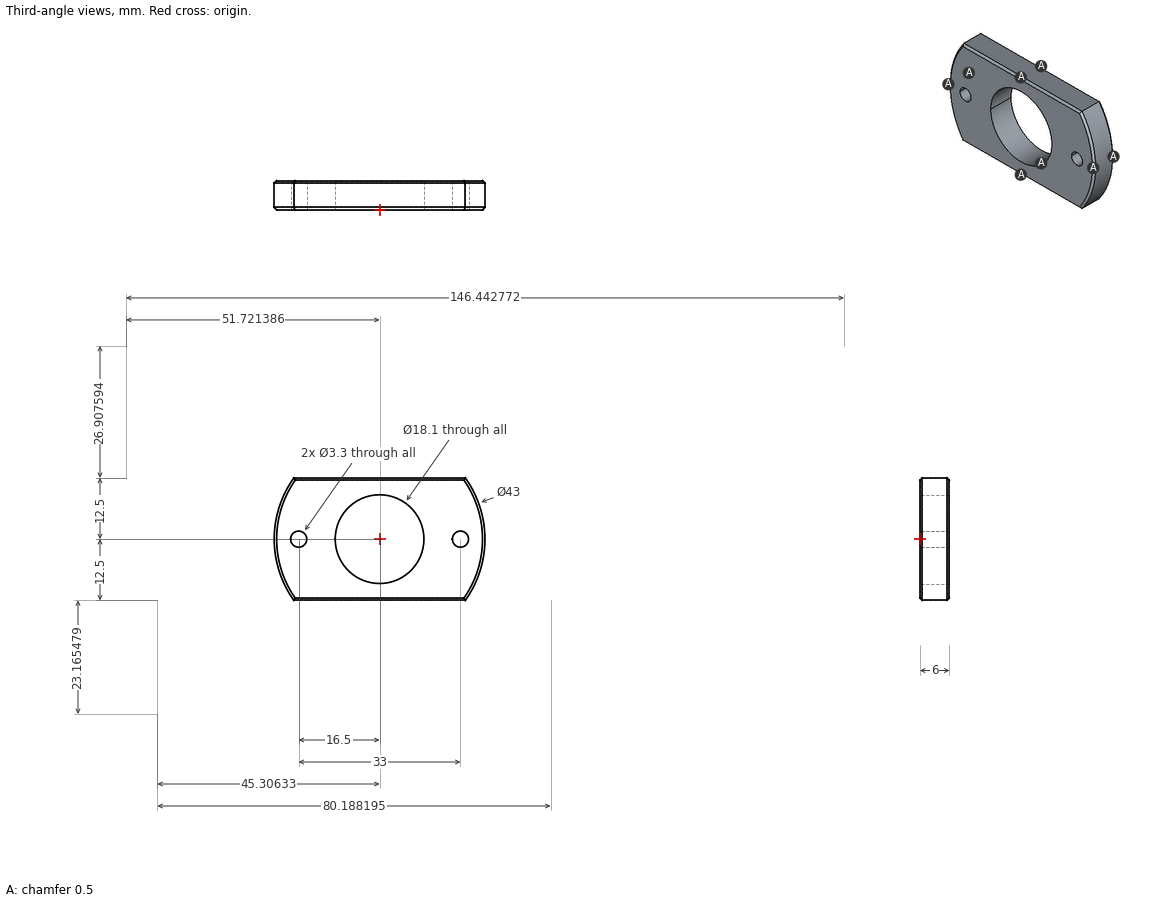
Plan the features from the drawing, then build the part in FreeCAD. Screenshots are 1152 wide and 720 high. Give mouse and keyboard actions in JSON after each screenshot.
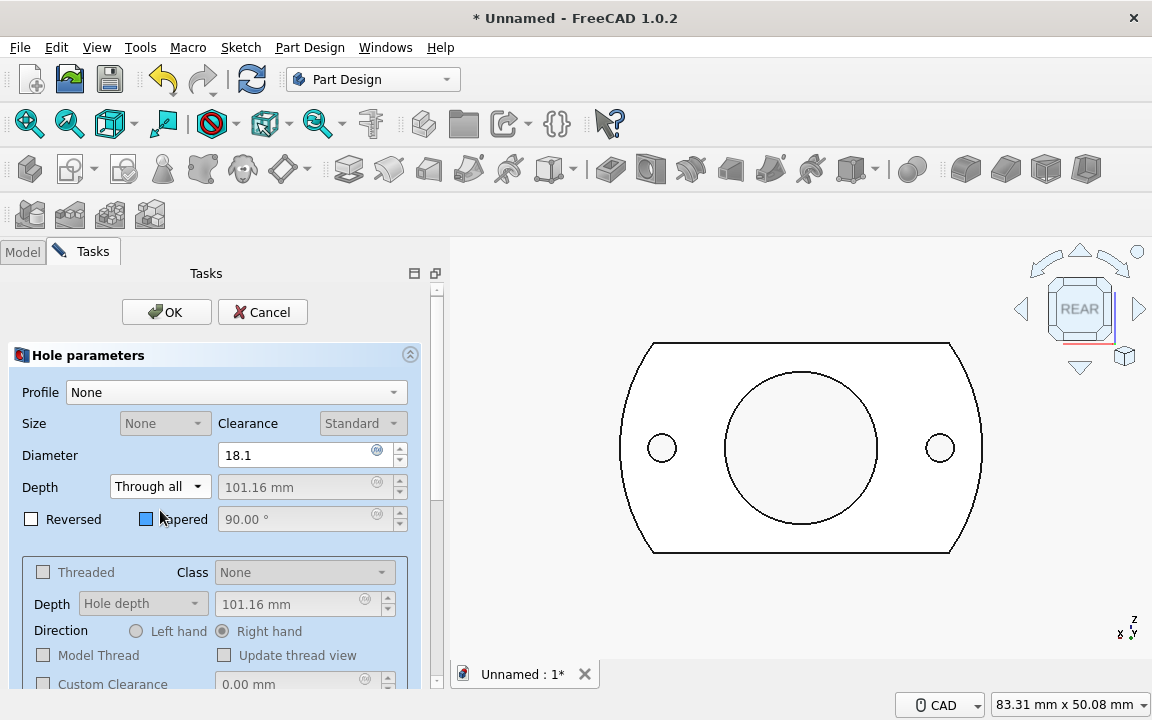
{"action": "left_click", "coordinate": [167, 312]}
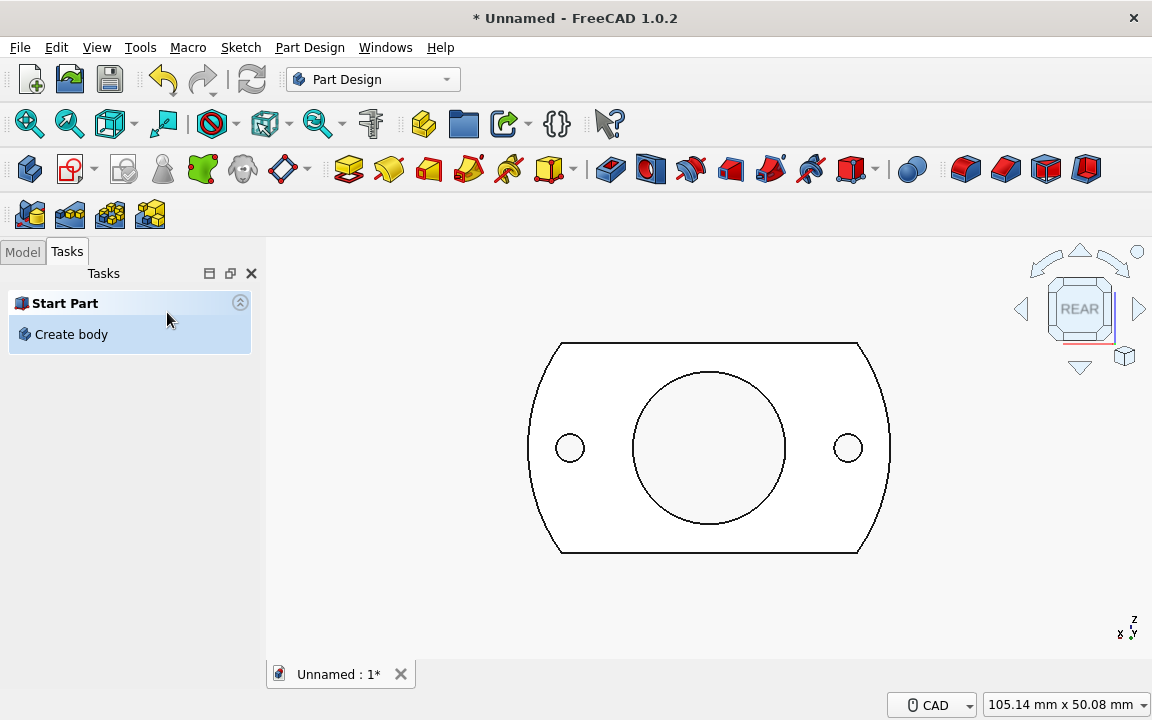
{"action": "left_click", "coordinate": [890, 447]}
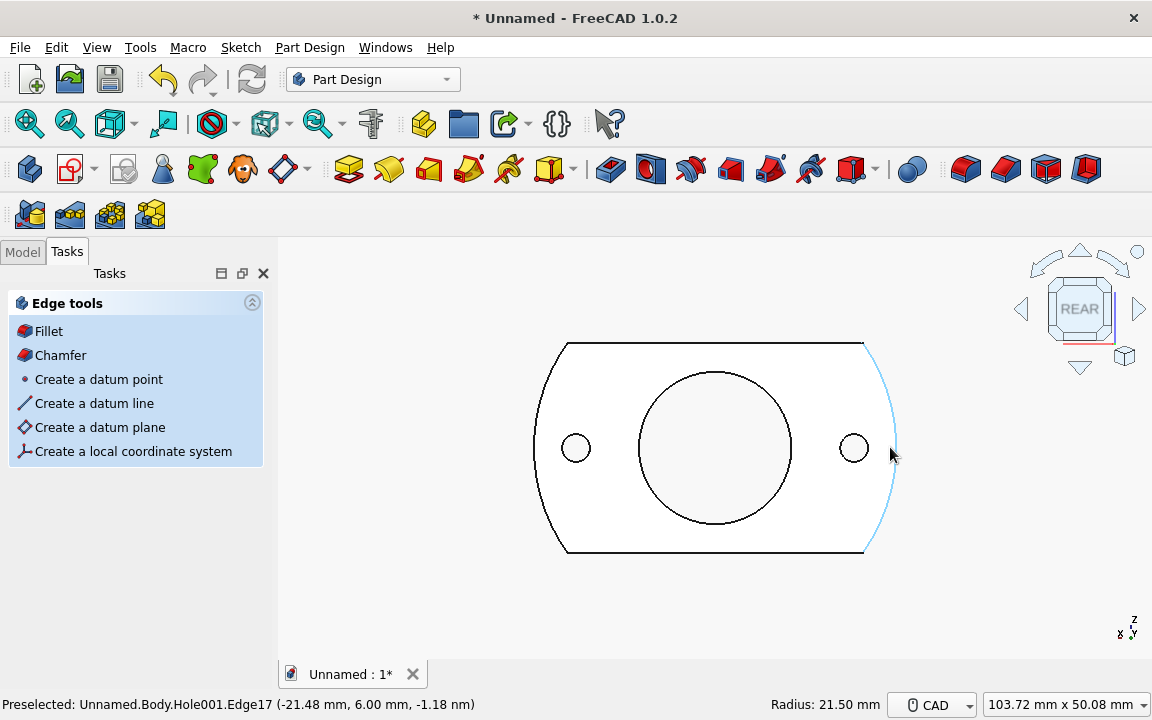
{"action": "left_click", "coordinate": [715, 552], "text": "ctrl"}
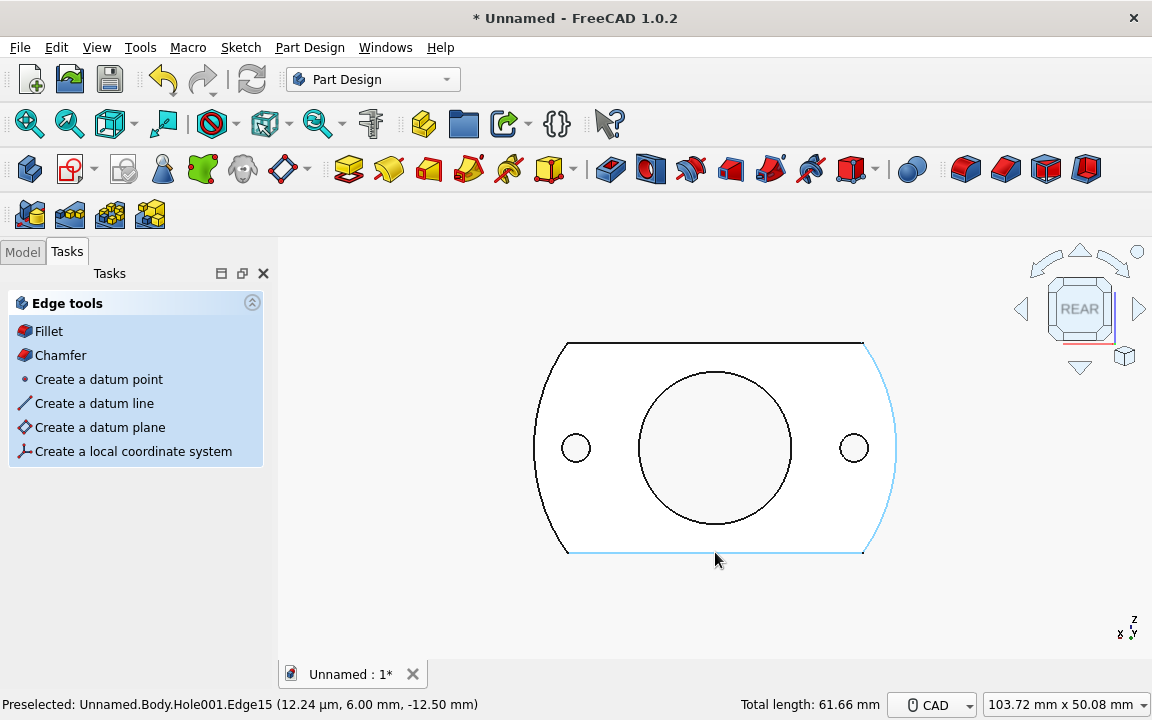
{"action": "left_click", "coordinate": [539, 492], "text": "ctrl"}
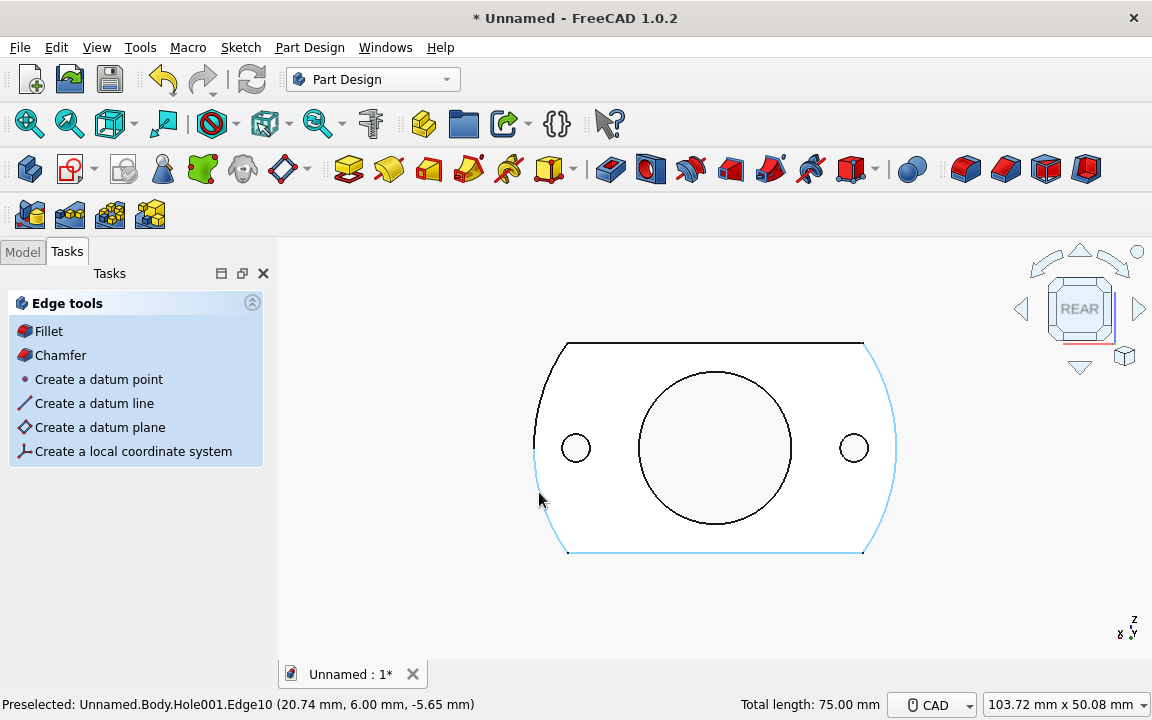
{"action": "key", "text": "0"}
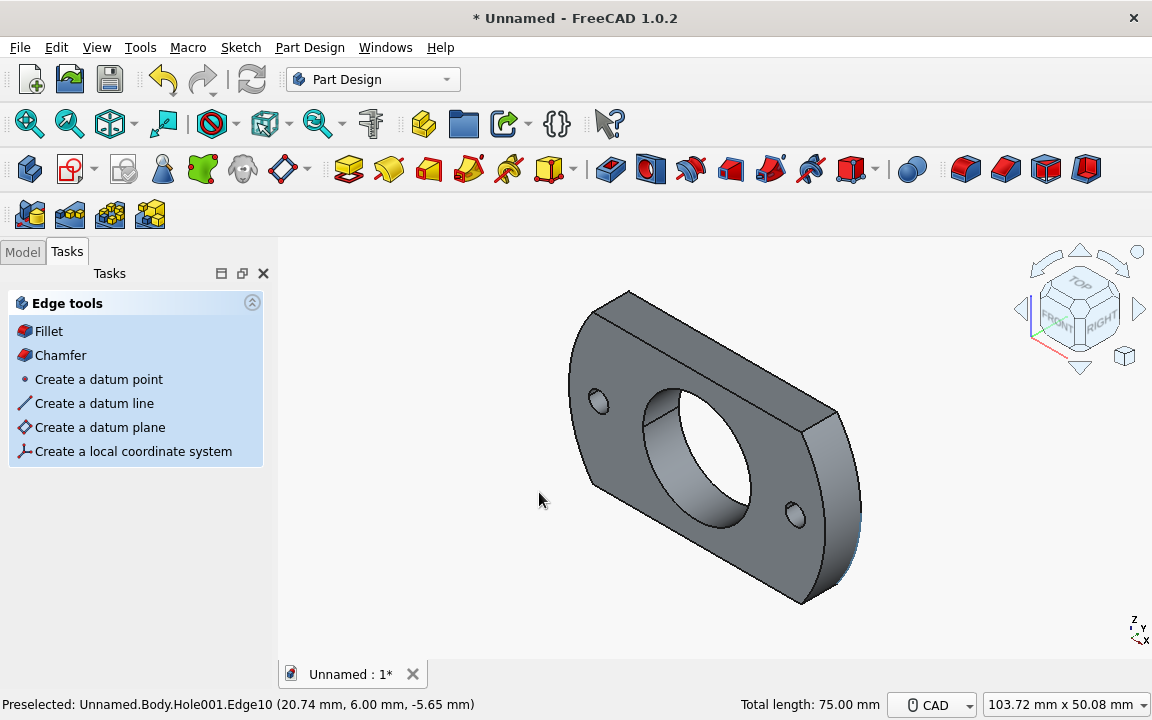
{"action": "left_click", "coordinate": [819, 483], "text": "ctrl"}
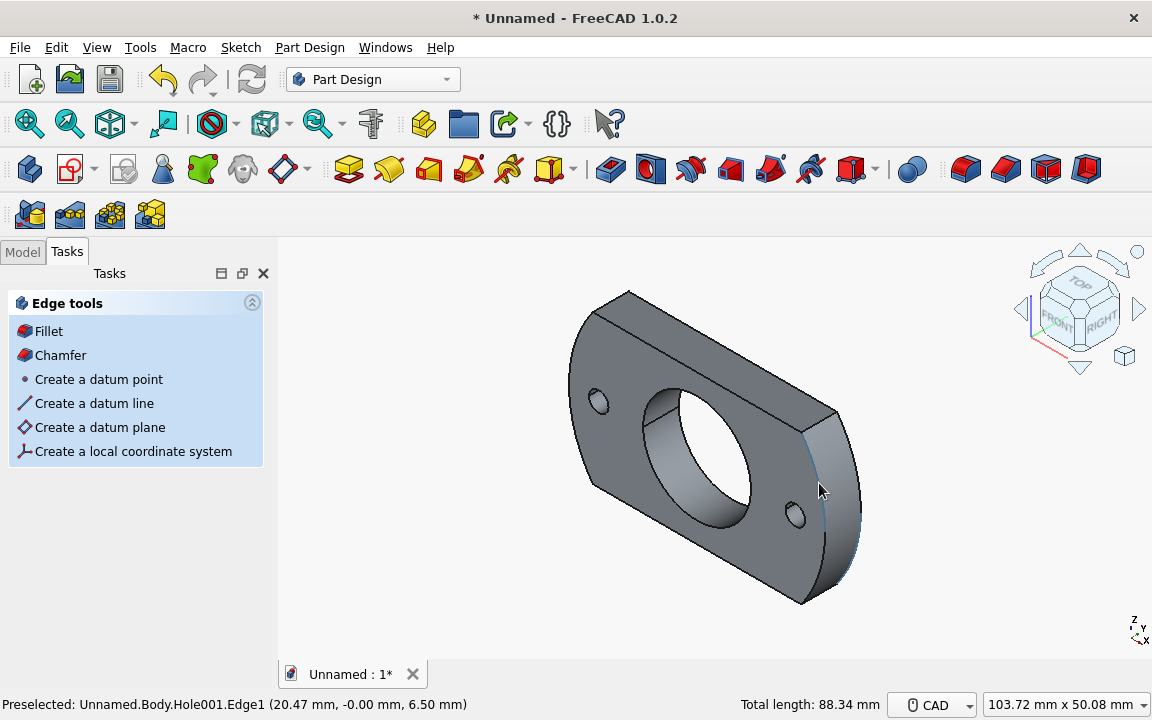
{"action": "left_click", "coordinate": [697, 371], "text": "ctrl"}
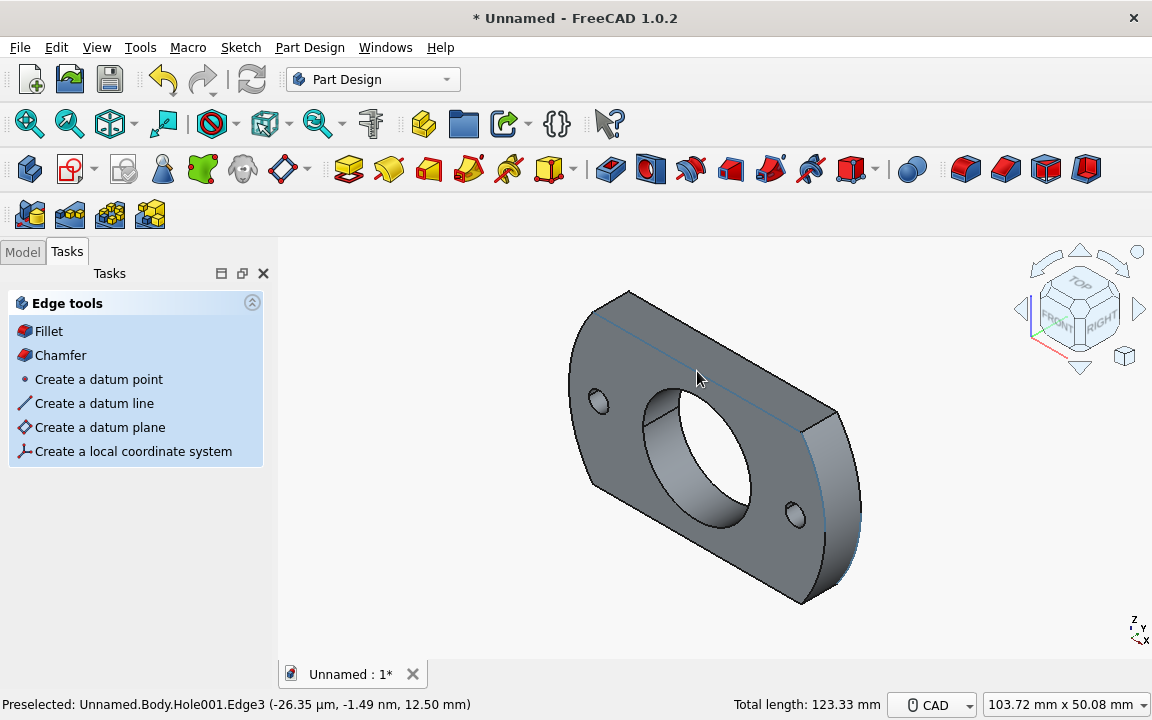
{"action": "key", "text": "2"}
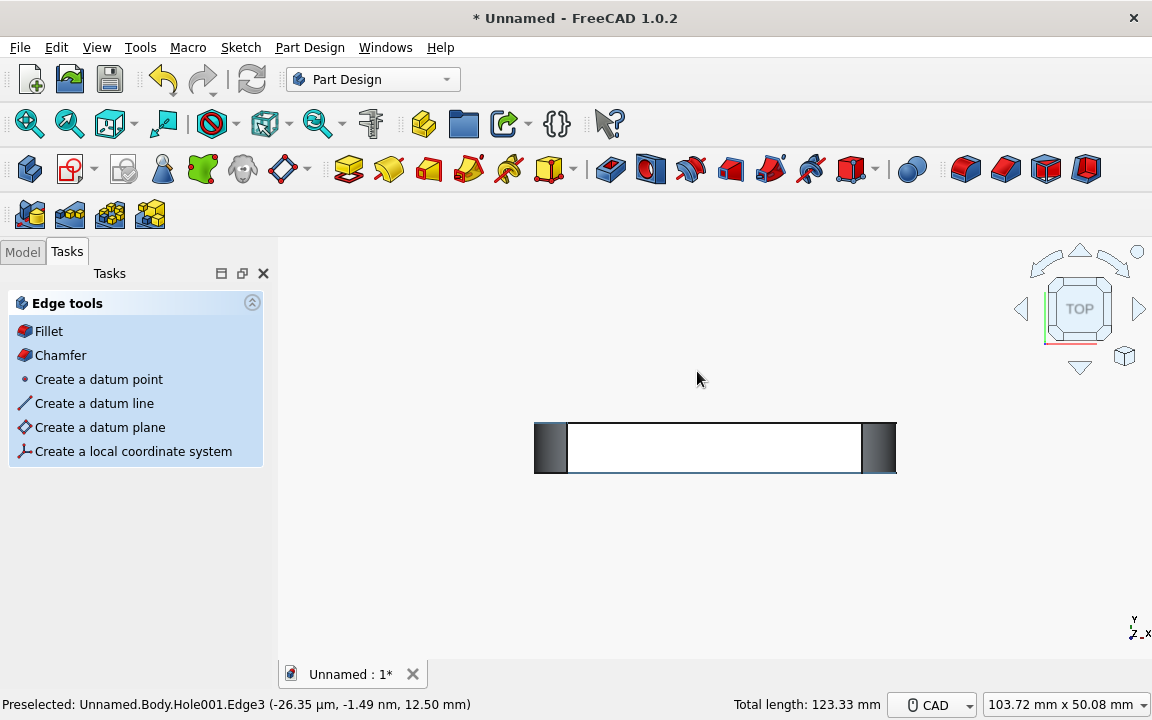
{"action": "left_click", "coordinate": [30, 124]}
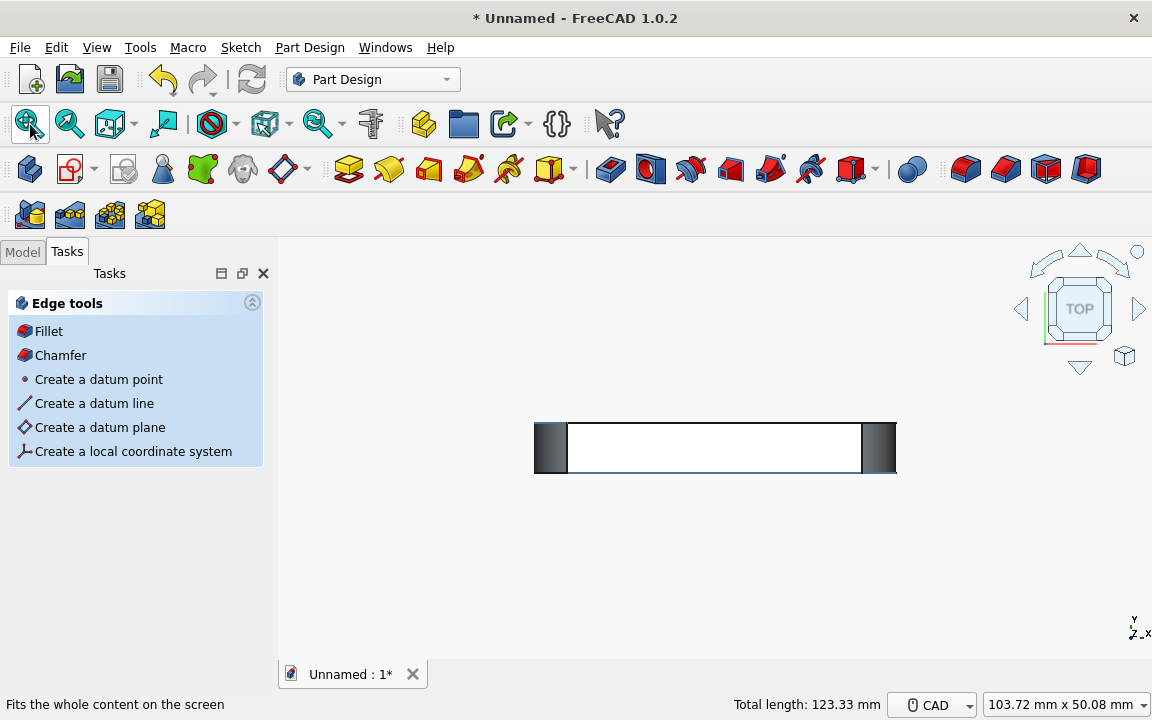
{"action": "left_click", "coordinate": [715, 422], "text": "ctrl"}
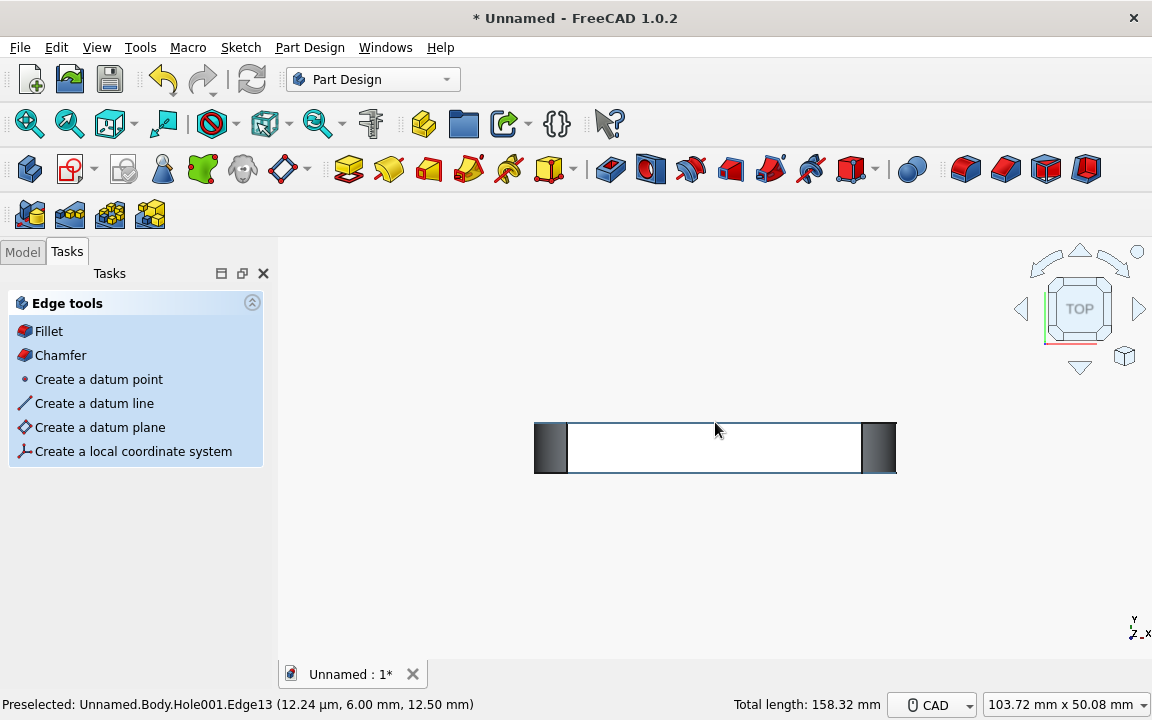
{"action": "key", "text": "1"}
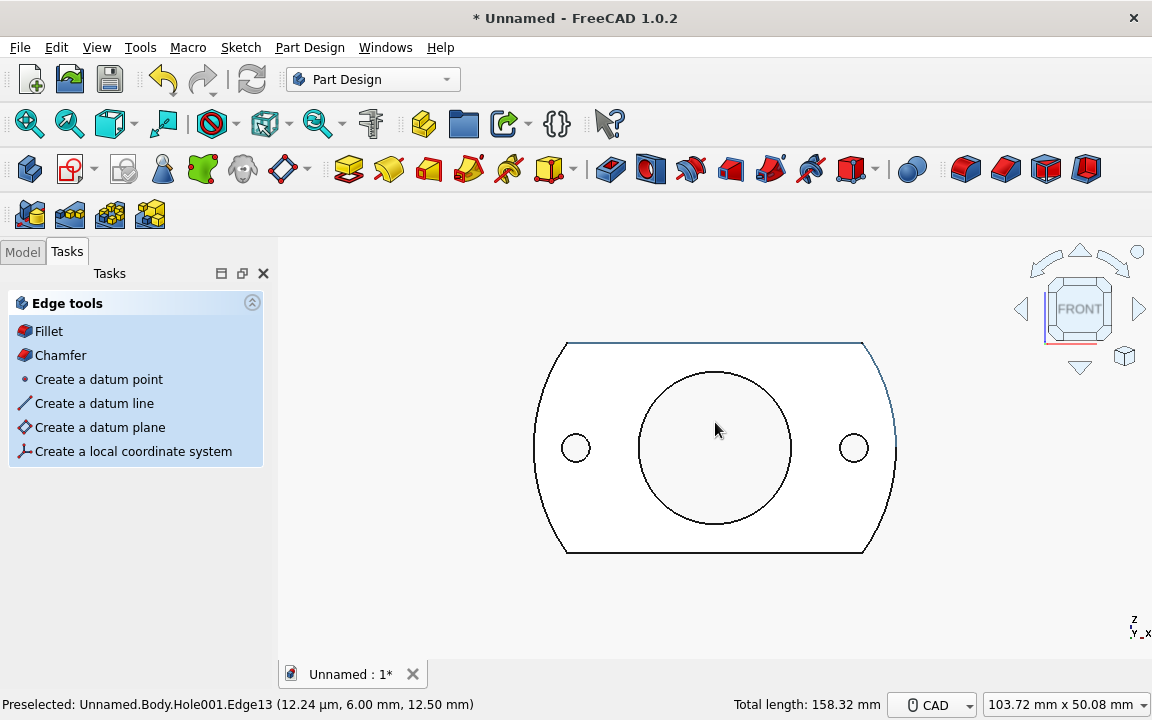
{"action": "left_click", "coordinate": [535, 425], "text": "ctrl"}